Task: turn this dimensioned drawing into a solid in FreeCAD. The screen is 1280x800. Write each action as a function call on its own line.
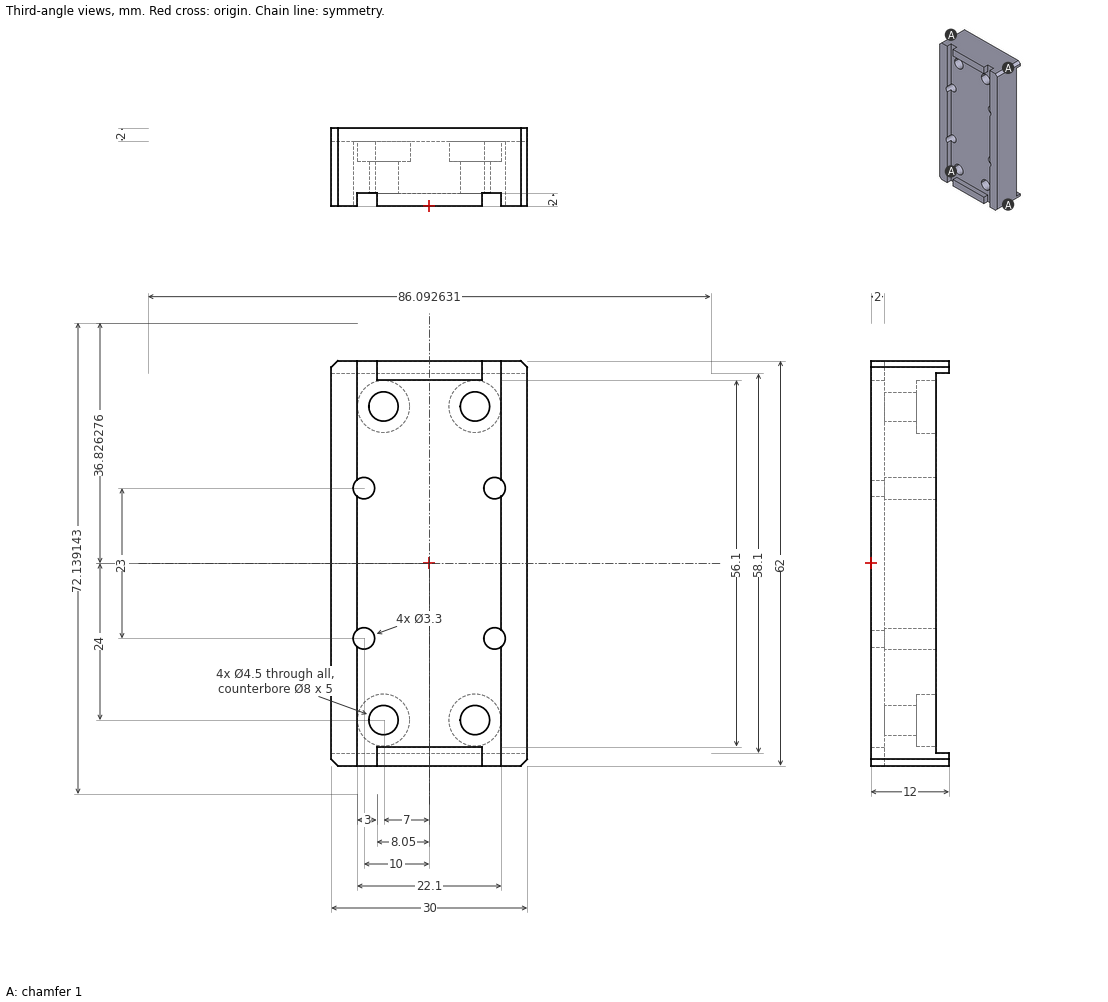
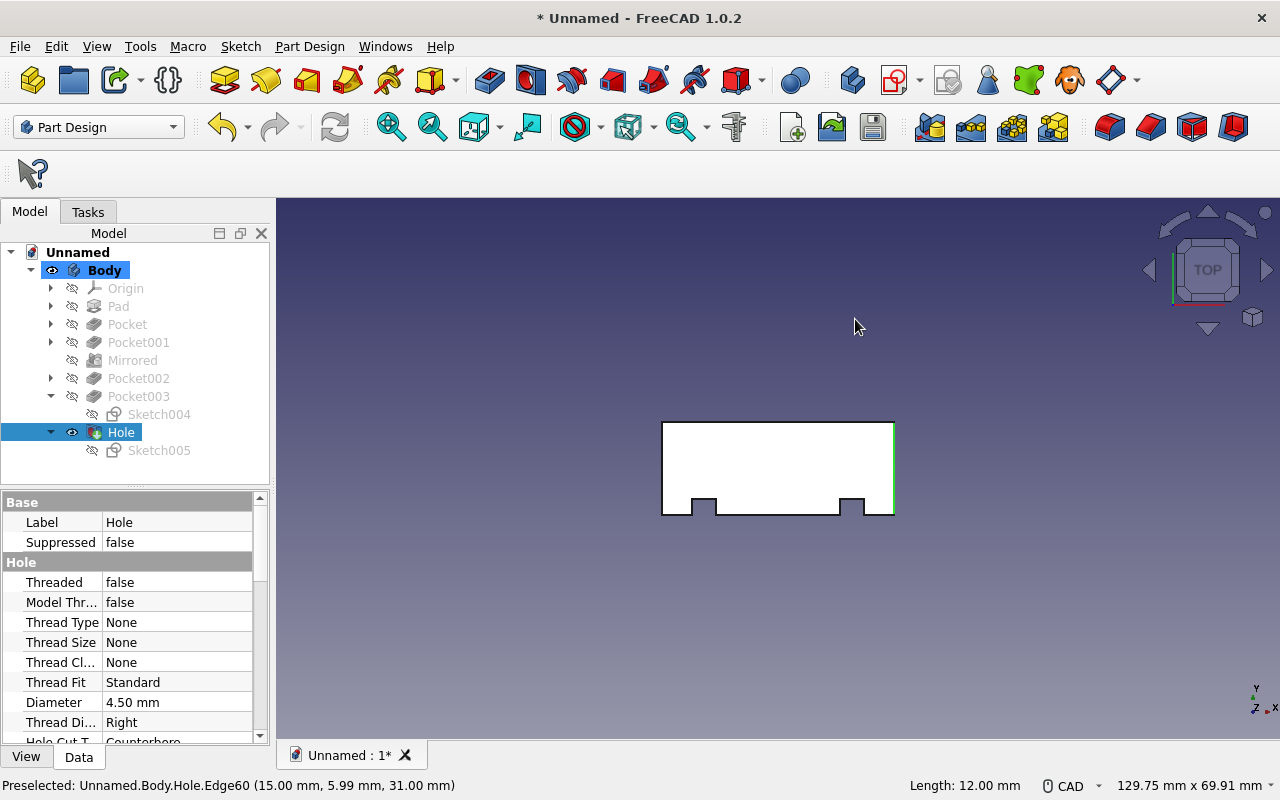
click(392, 128)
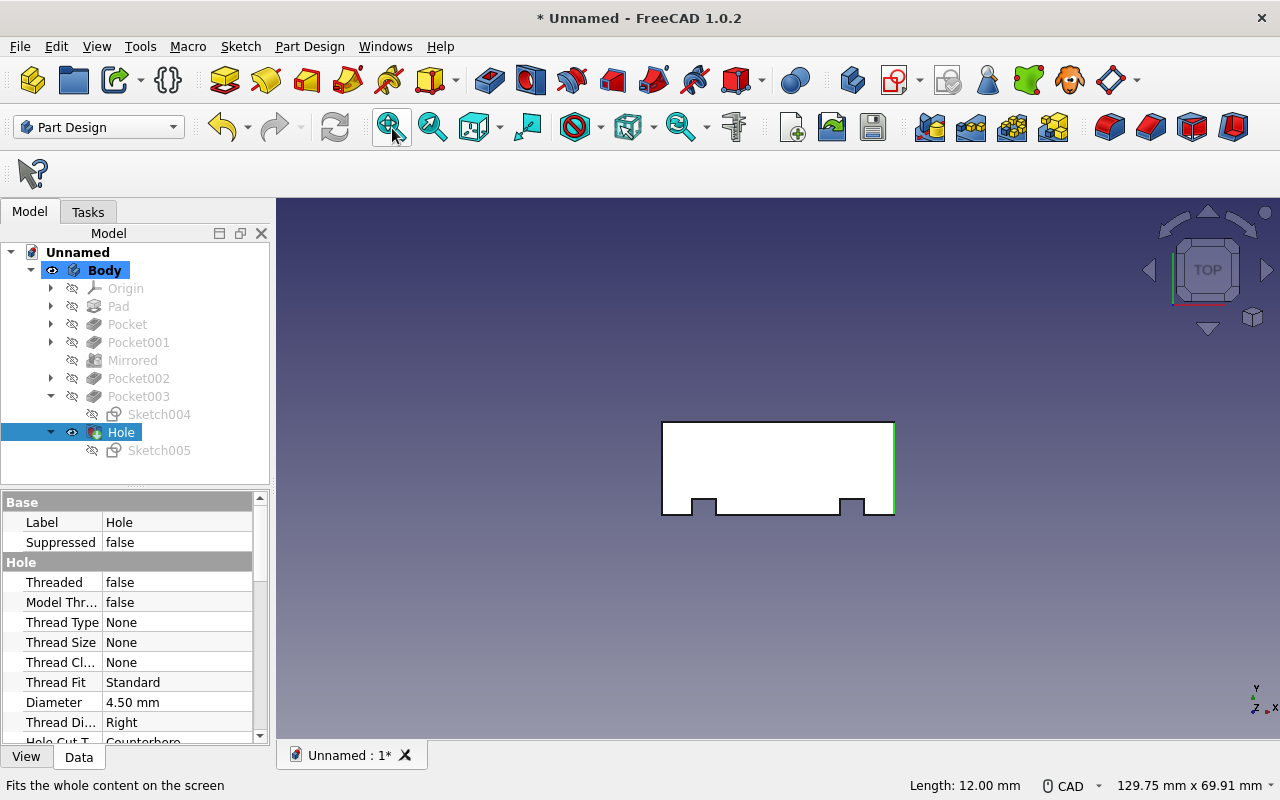
click(662, 467, ctrl)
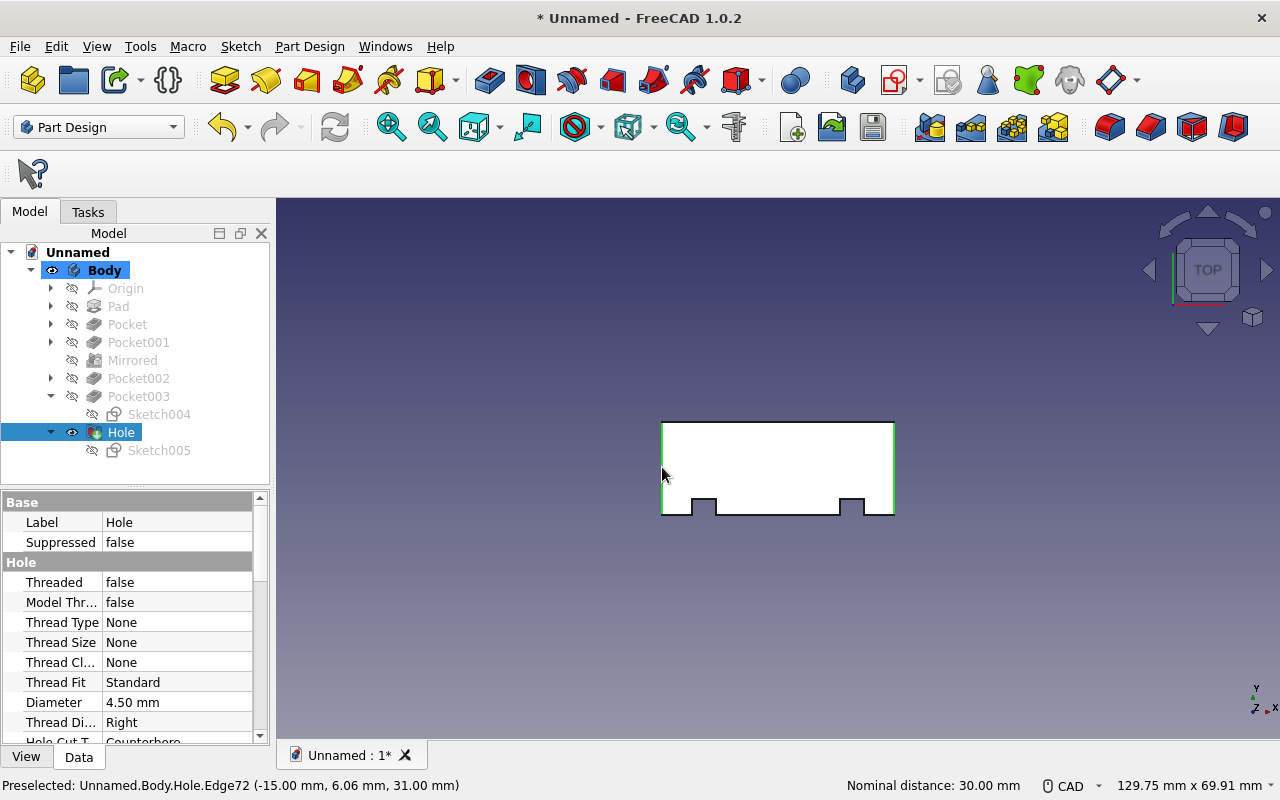
key(1)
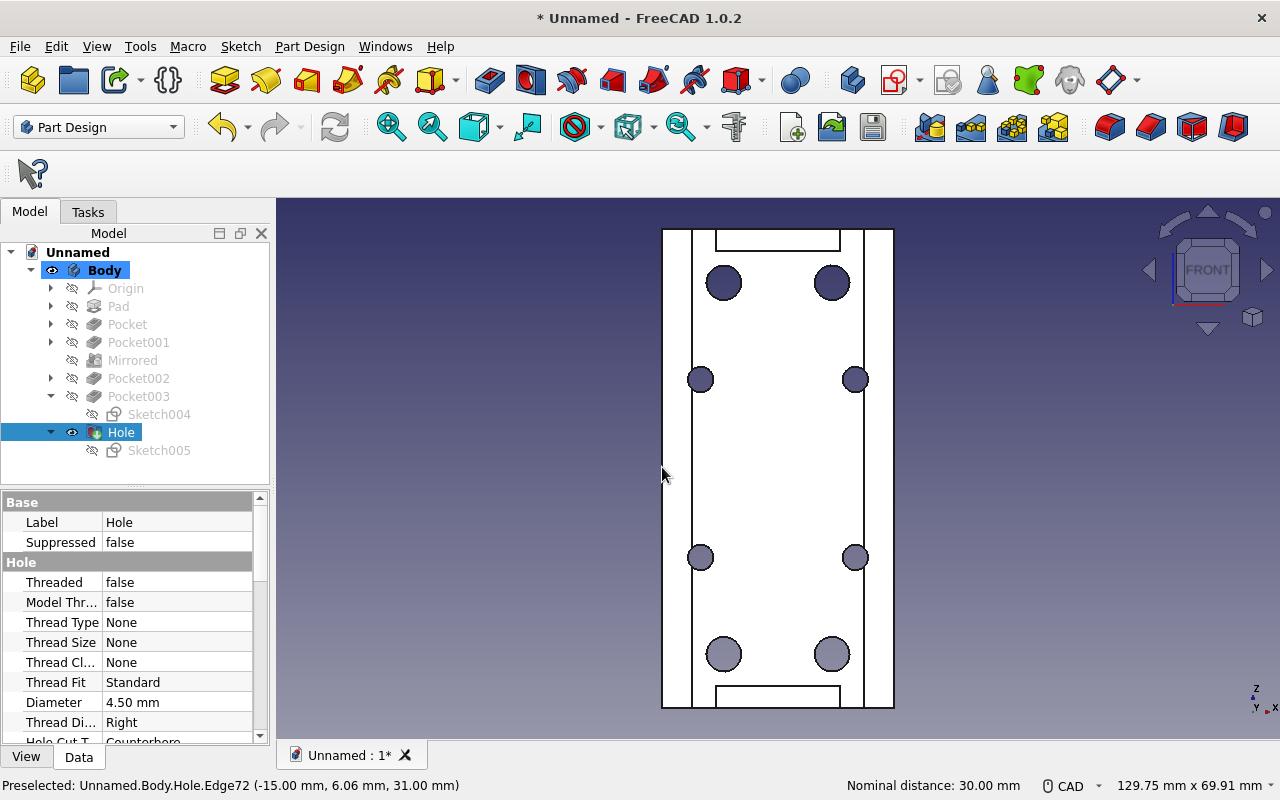
key(3)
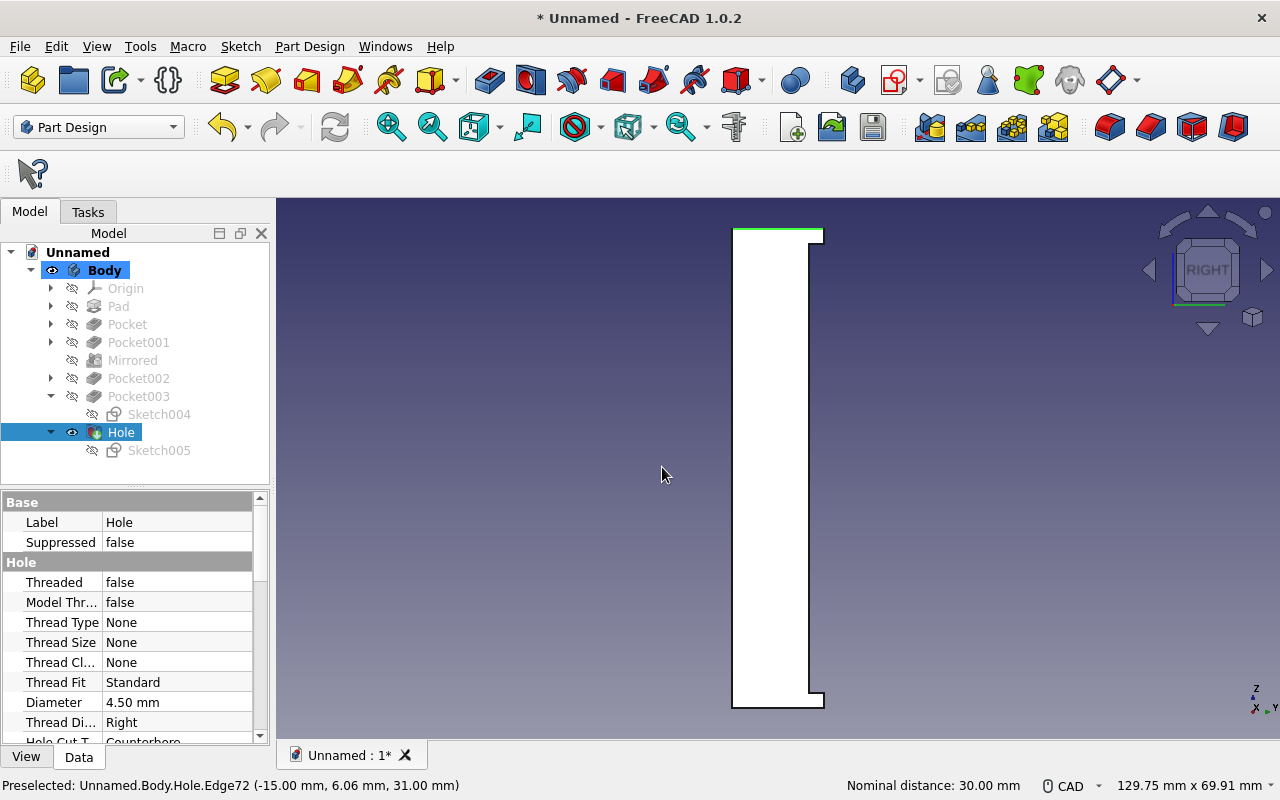
click(778, 707, ctrl)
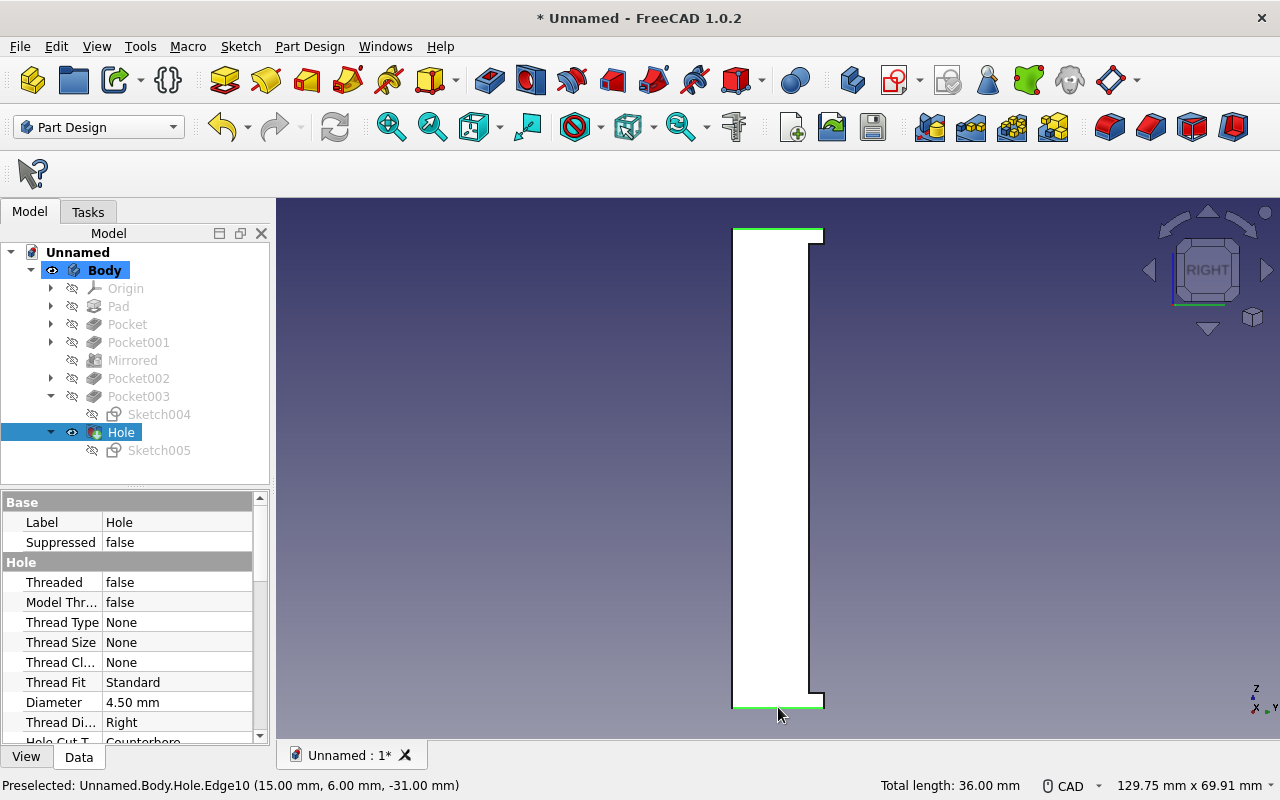
key(5)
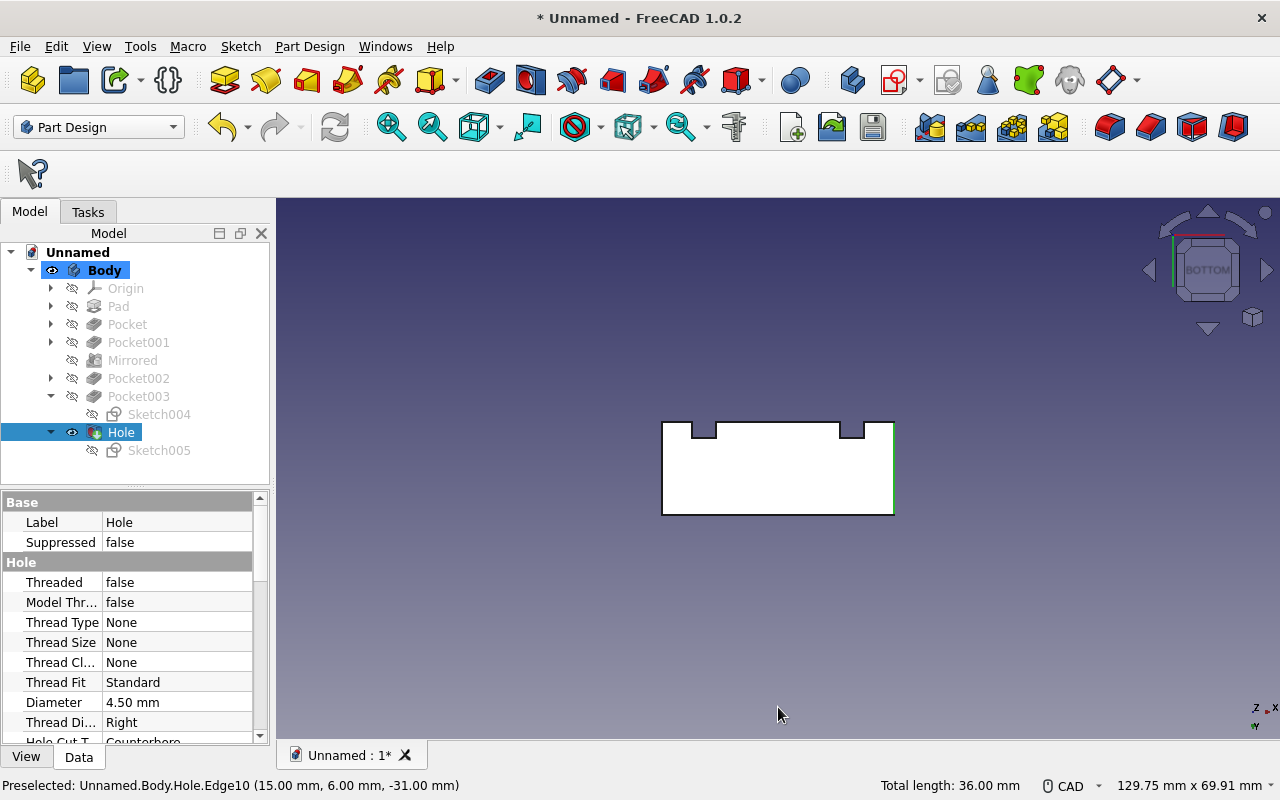
click(392, 128)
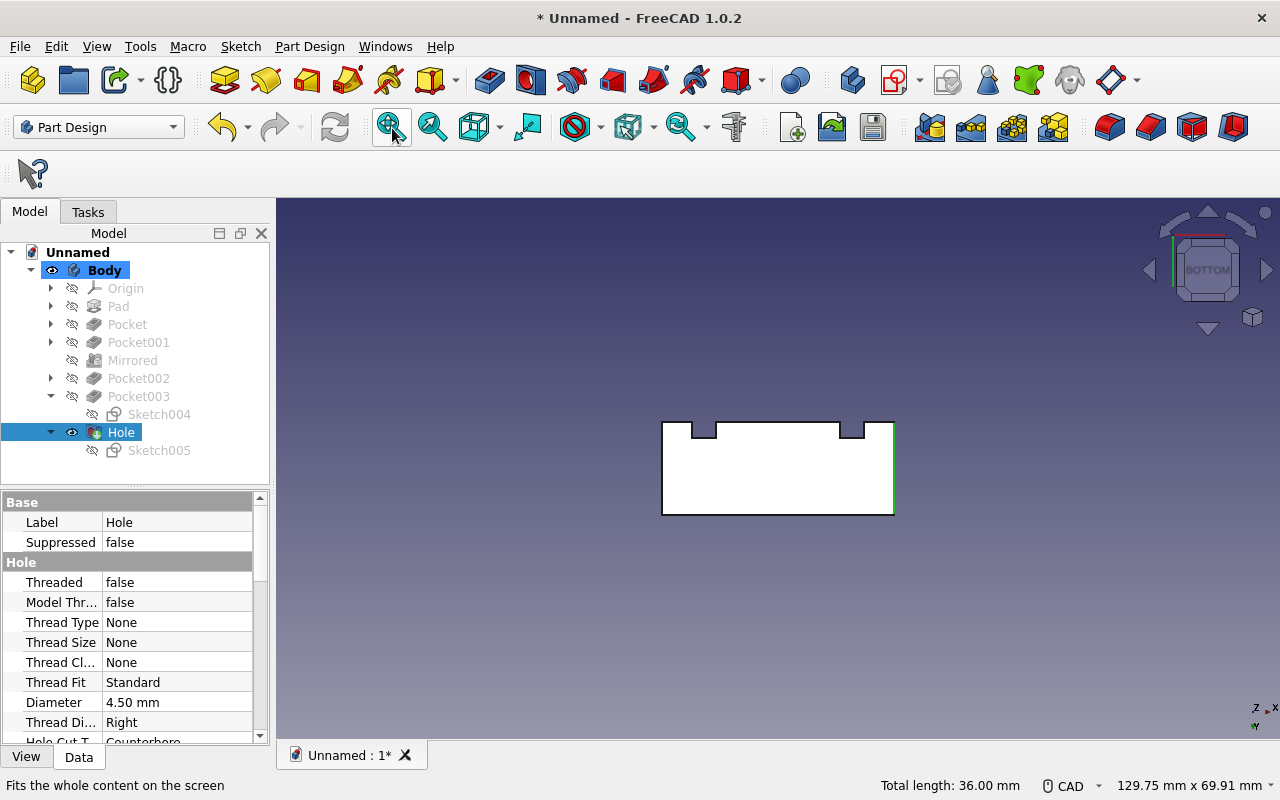
click(662, 467, ctrl)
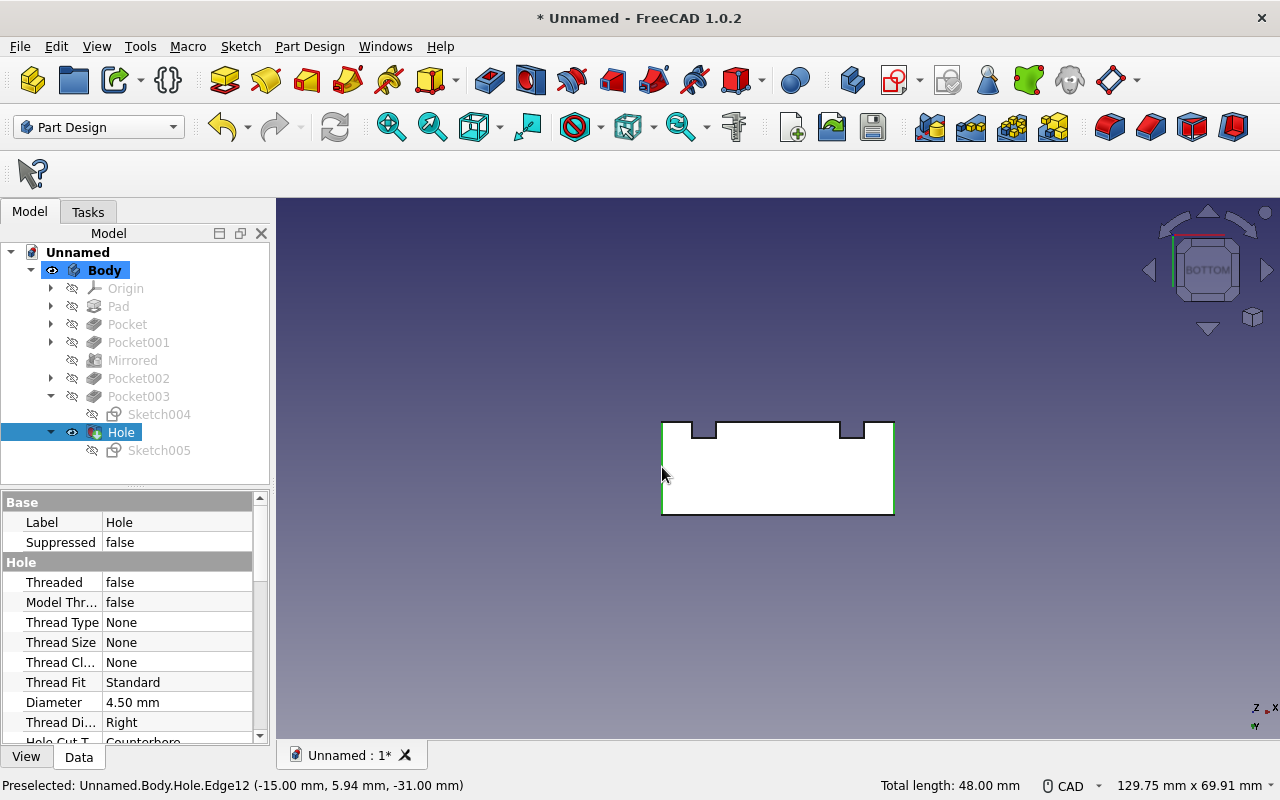
click(1151, 128)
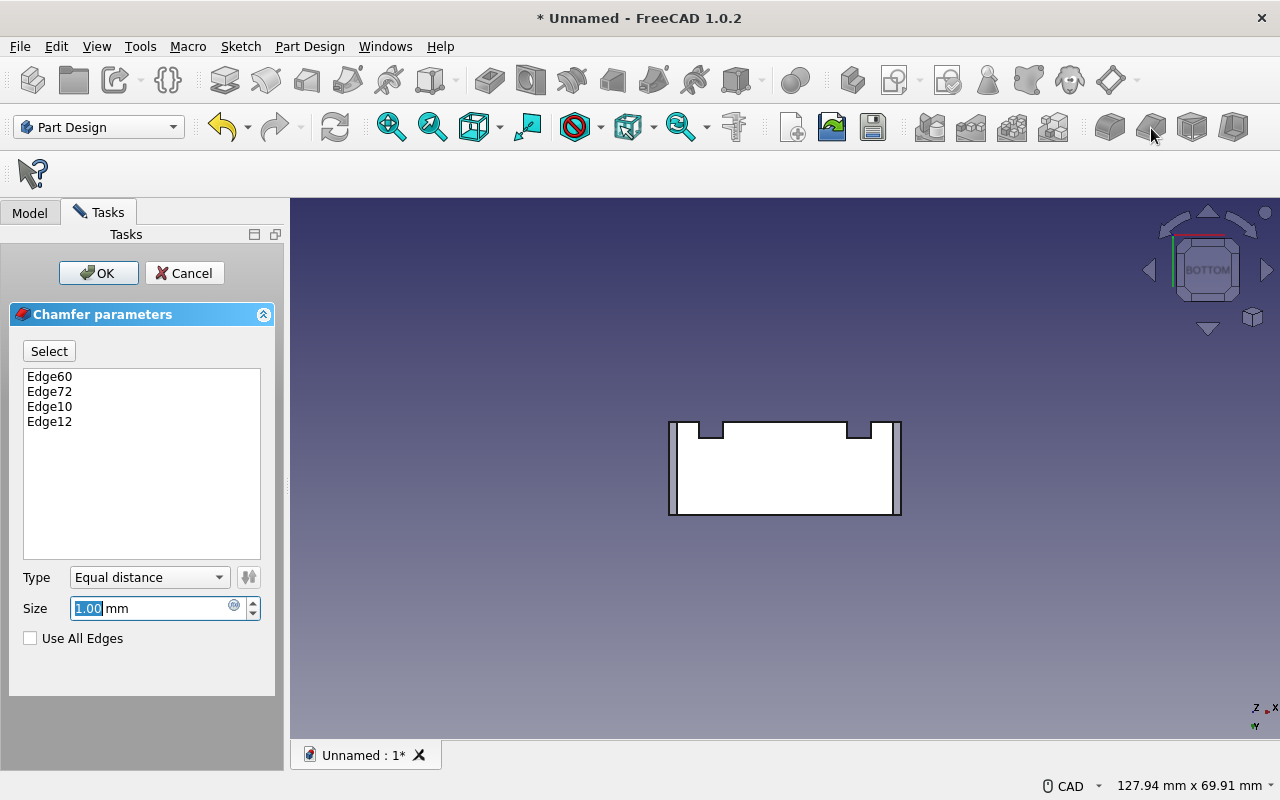
text(1)
key(Tab)